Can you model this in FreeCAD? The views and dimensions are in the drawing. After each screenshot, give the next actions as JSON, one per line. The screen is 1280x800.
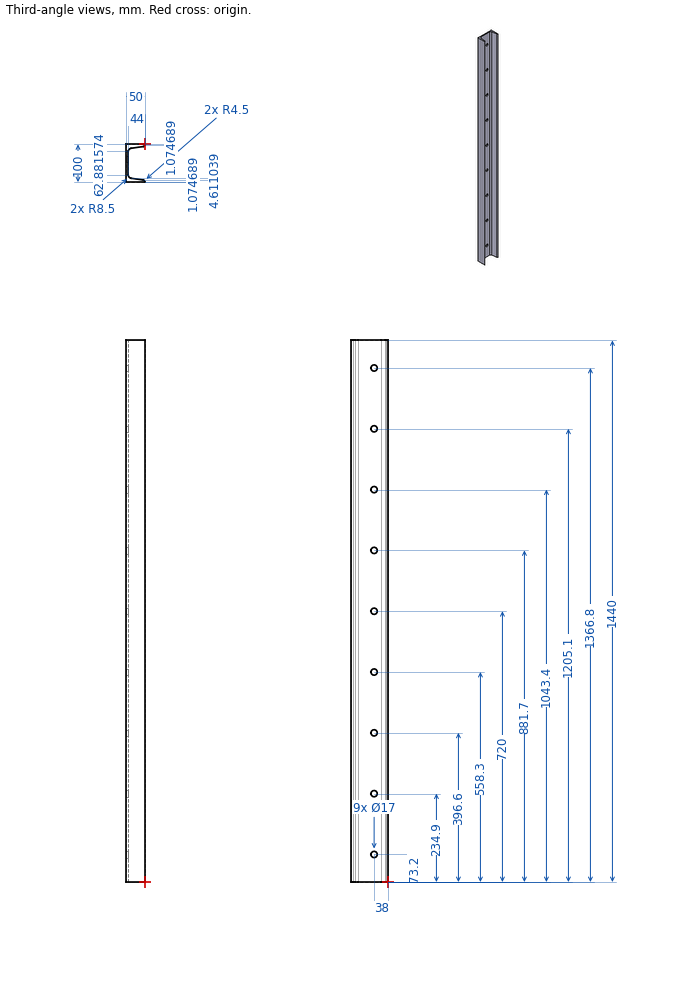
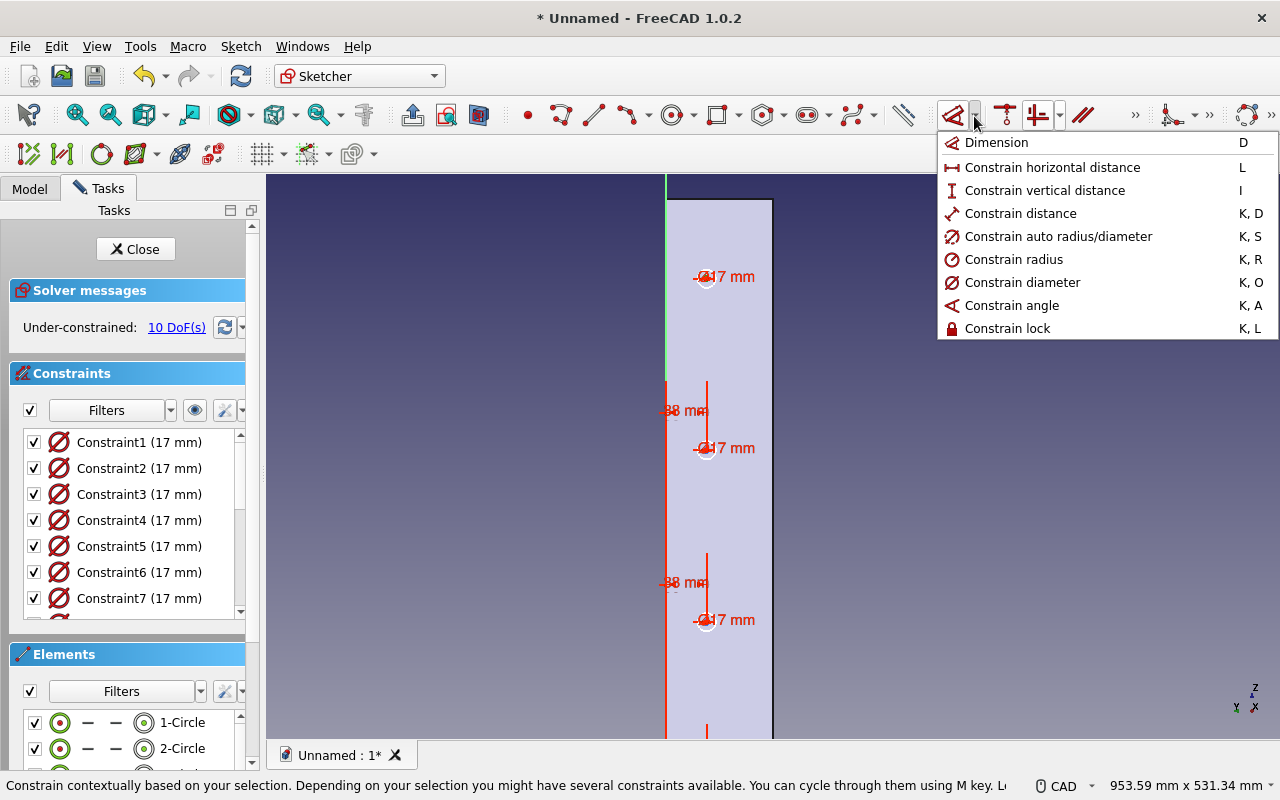
{"action": "left_click", "coordinate": [1108, 168]}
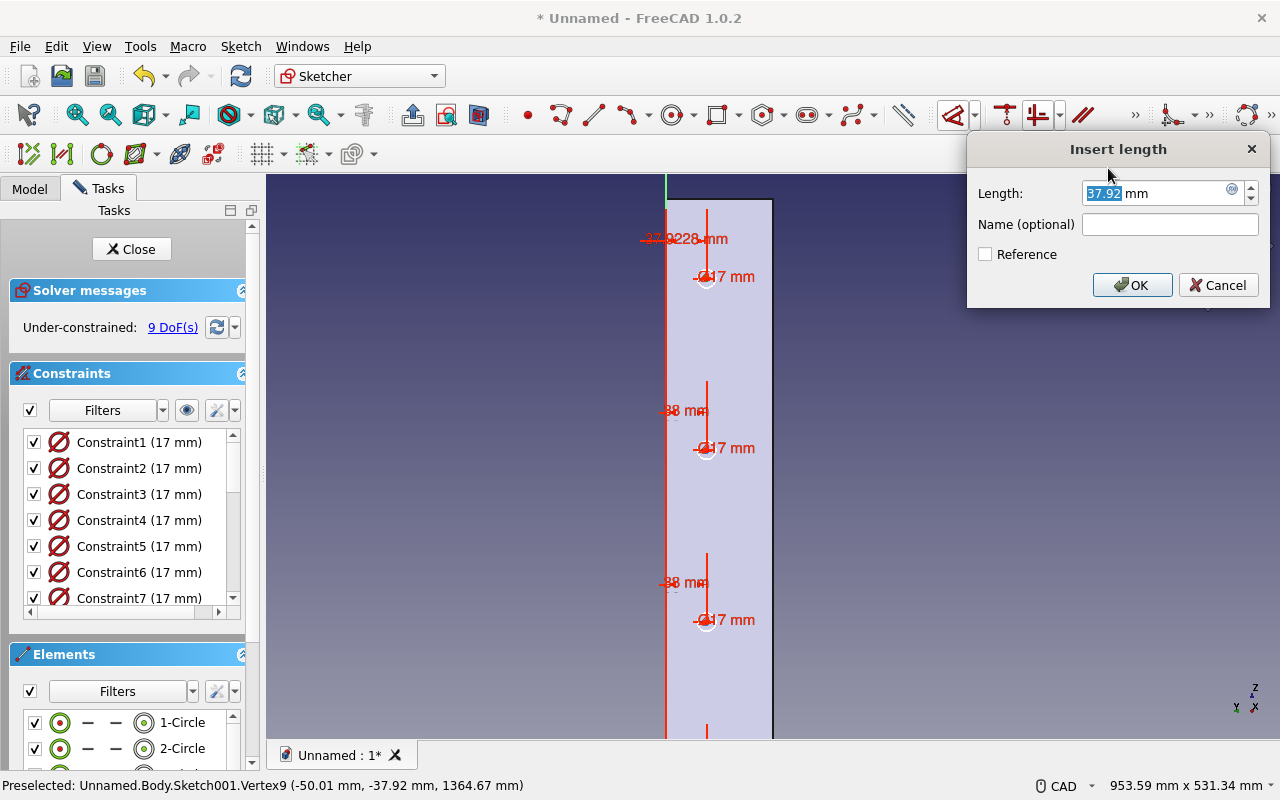
{"action": "type", "text": "38"}
{"action": "key", "text": "Return"}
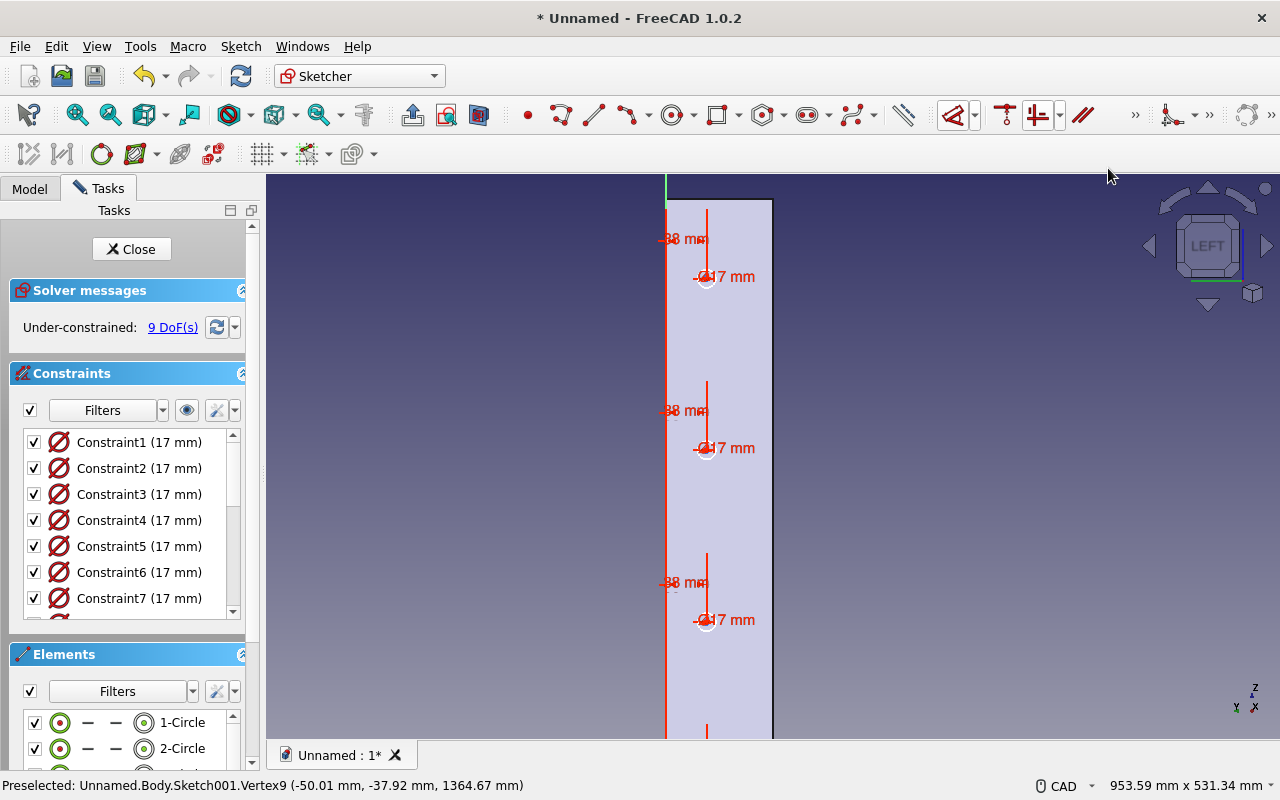
{"action": "scroll", "coordinate": [709, 279], "scroll_direction": "down", "scroll_amount": 7}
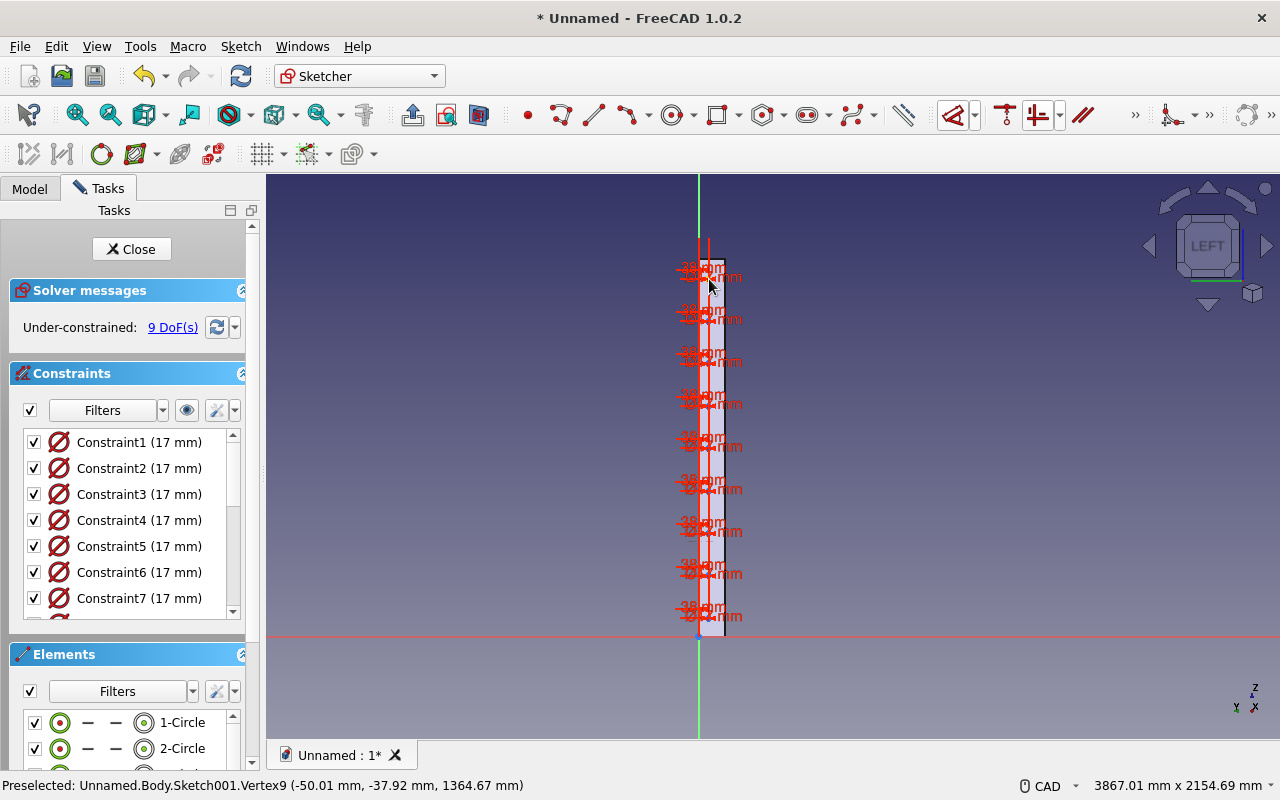
{"action": "left_click", "coordinate": [709, 448]}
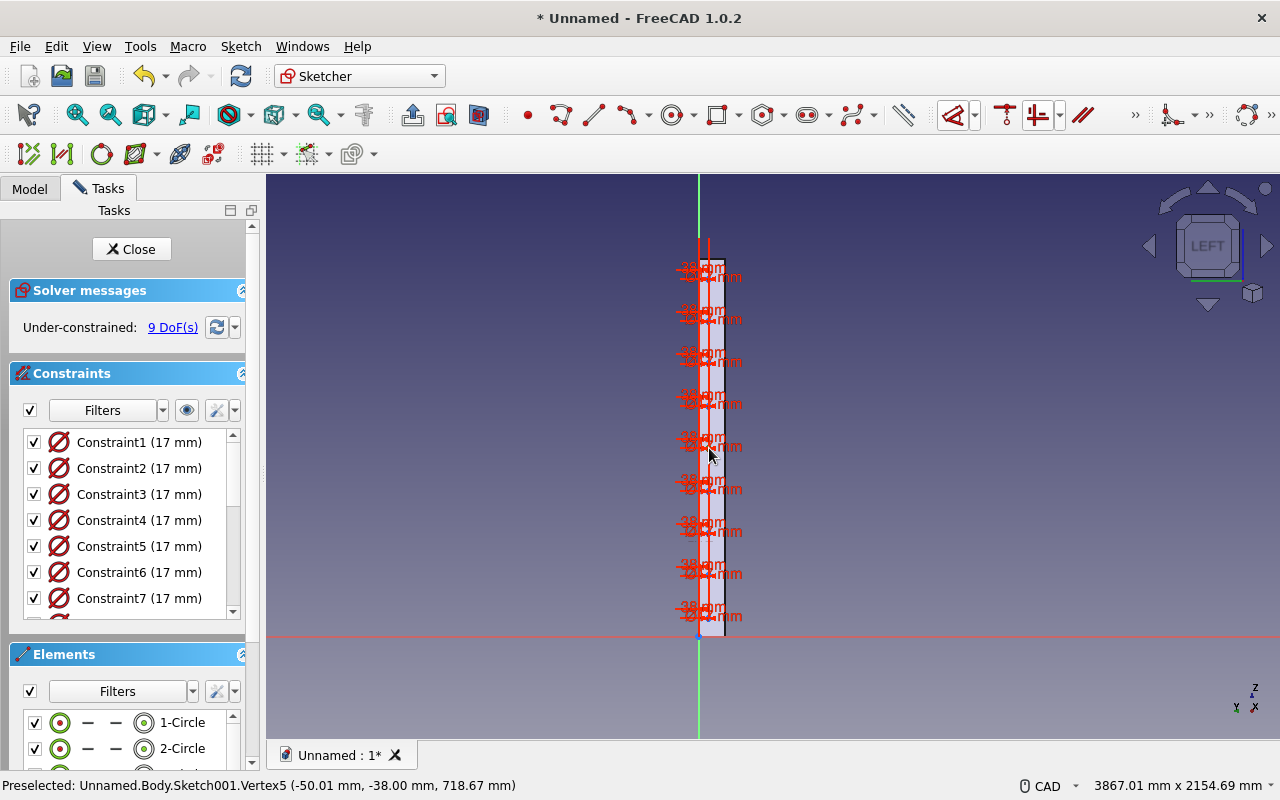
{"action": "left_click", "coordinate": [974, 116]}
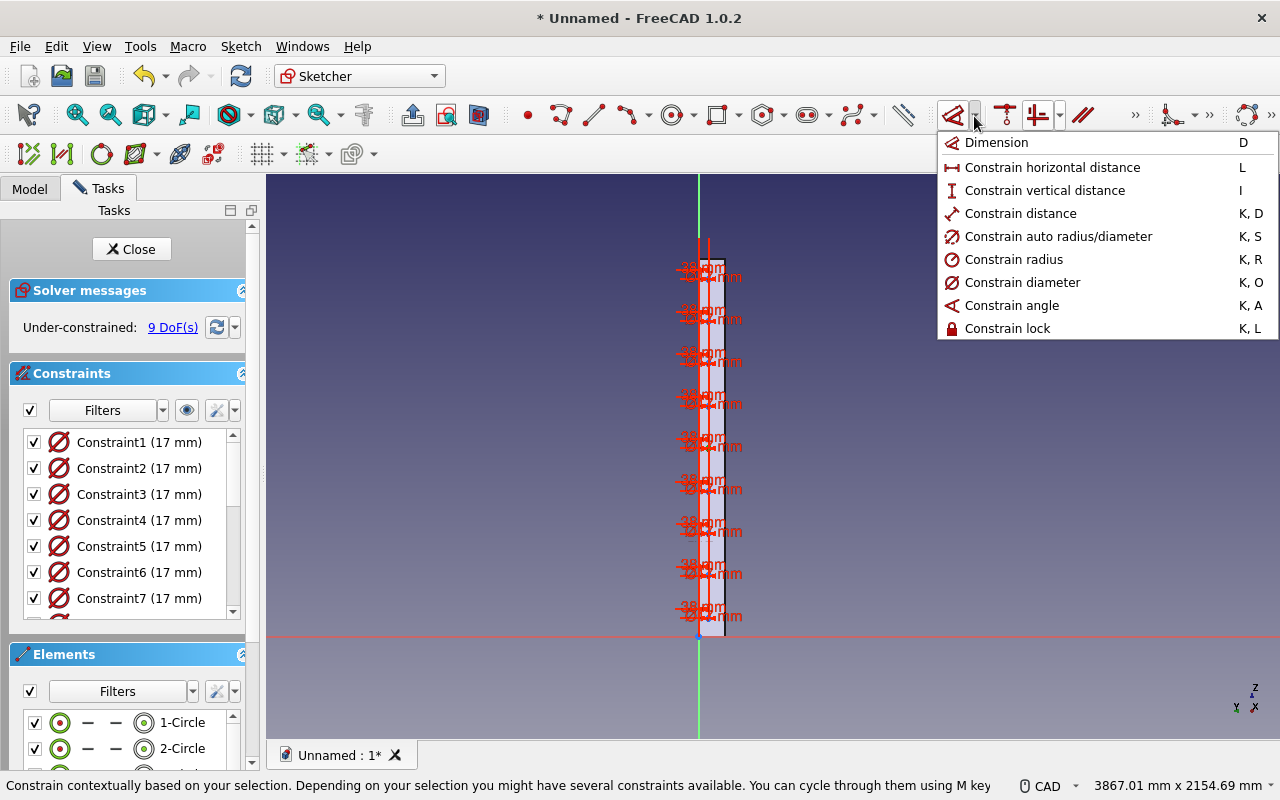
{"action": "left_click", "coordinate": [1108, 190]}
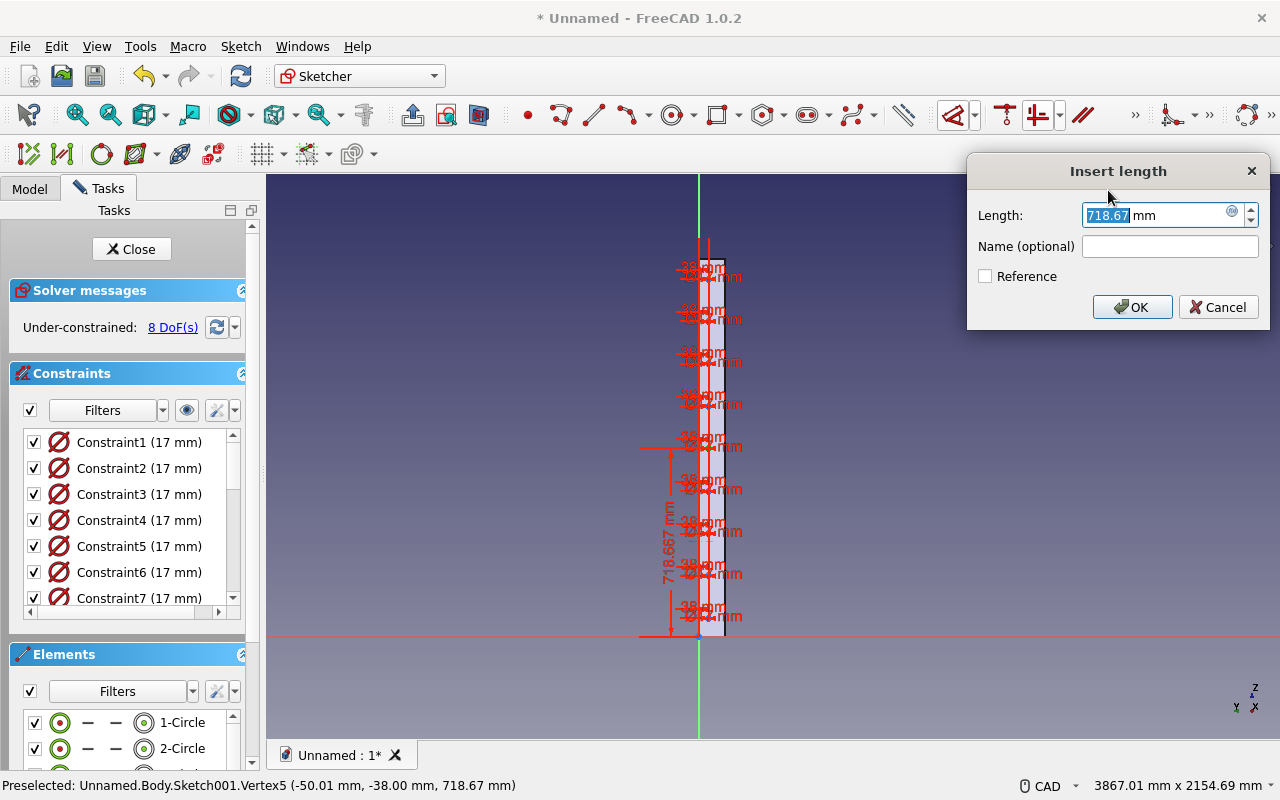
{"action": "type", "text": "720"}
{"action": "key", "text": "Return"}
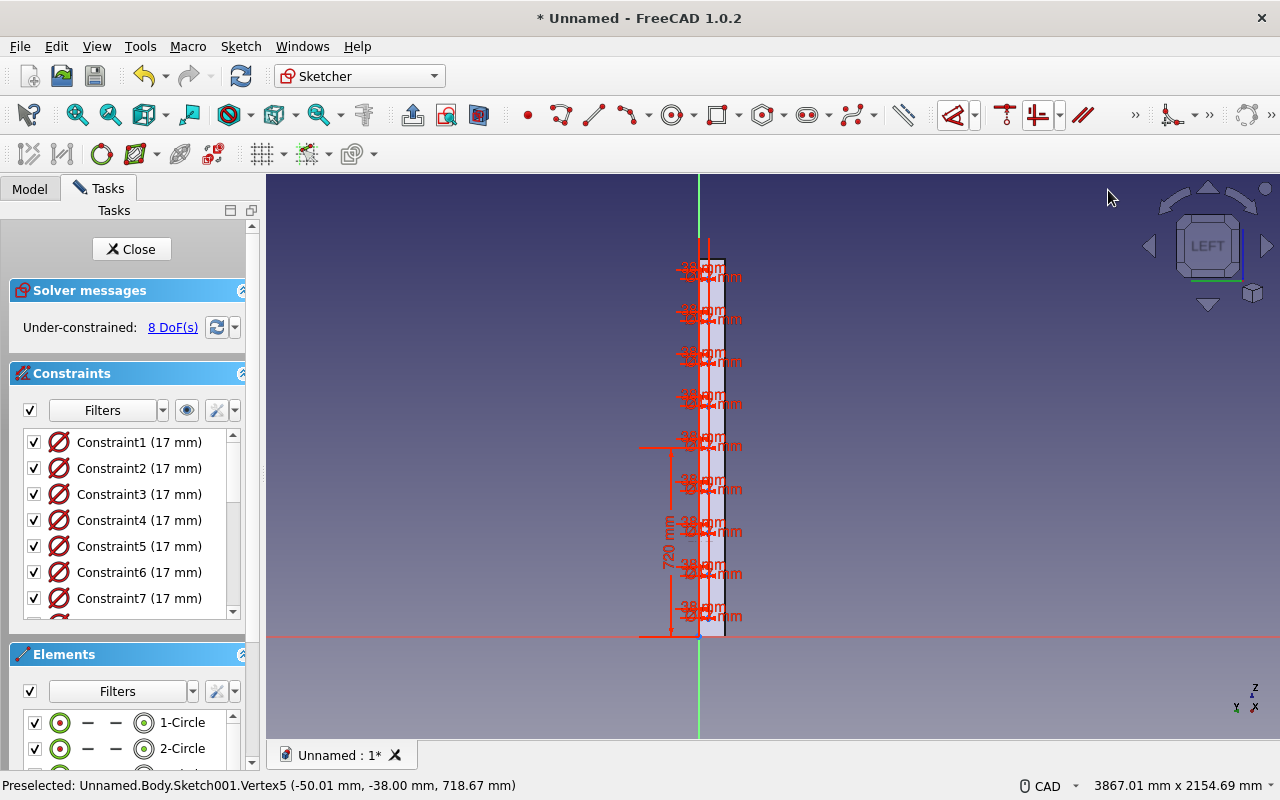
{"action": "scroll", "coordinate": [709, 618], "scroll_direction": "up", "scroll_amount": 4}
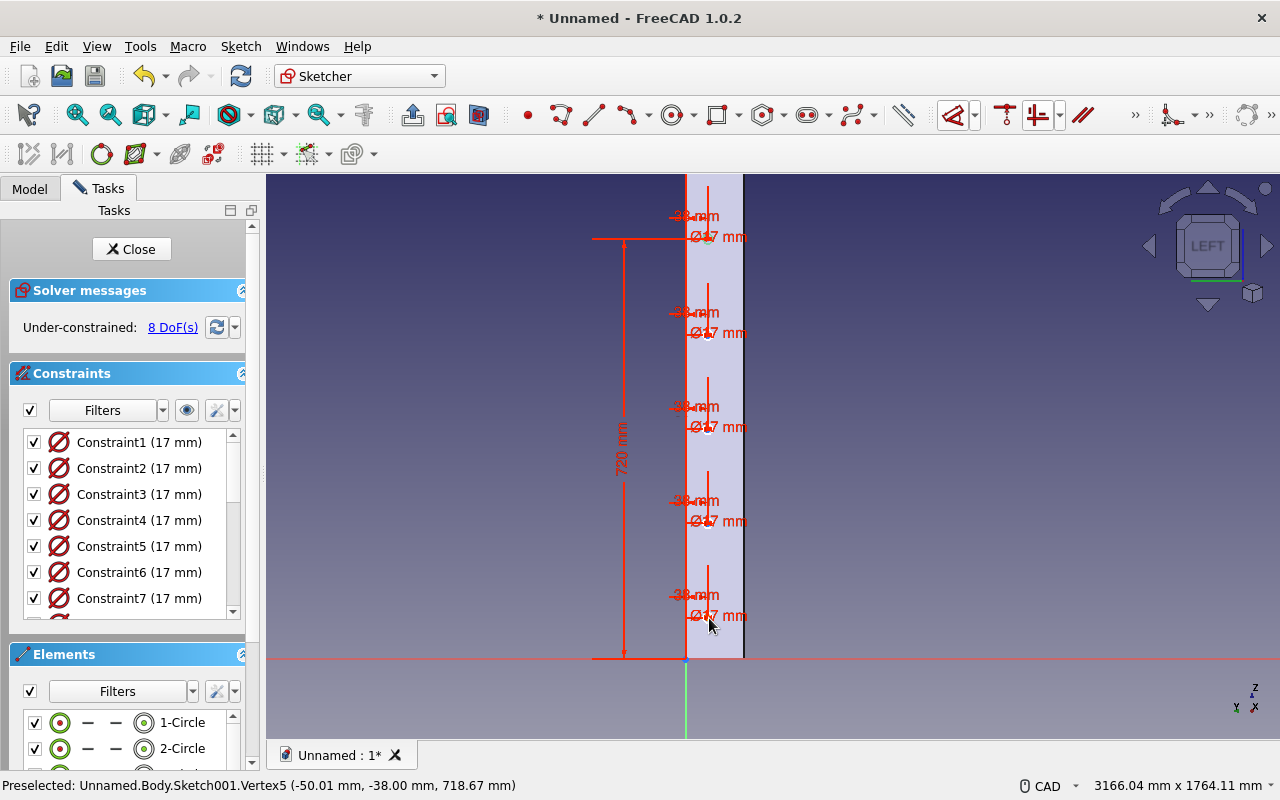
{"action": "left_click", "coordinate": [708, 618]}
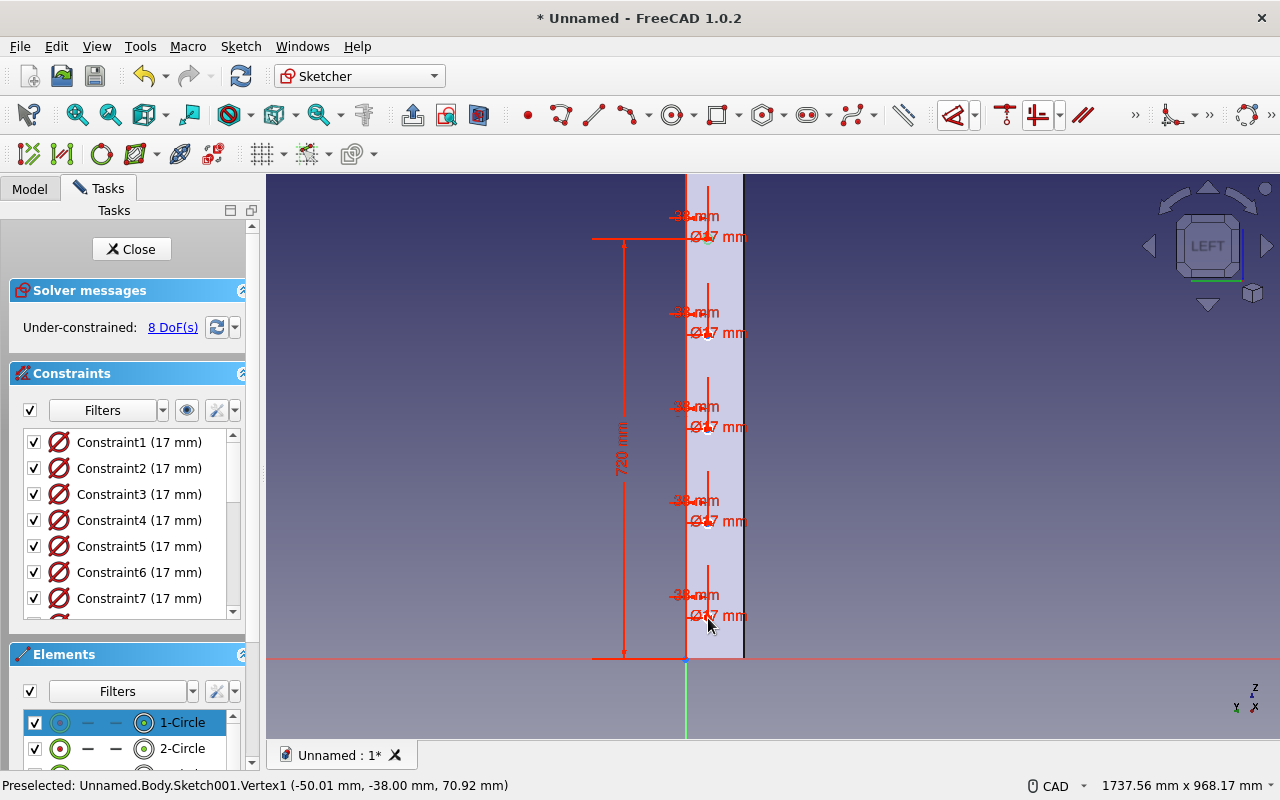
{"action": "left_click", "coordinate": [974, 116]}